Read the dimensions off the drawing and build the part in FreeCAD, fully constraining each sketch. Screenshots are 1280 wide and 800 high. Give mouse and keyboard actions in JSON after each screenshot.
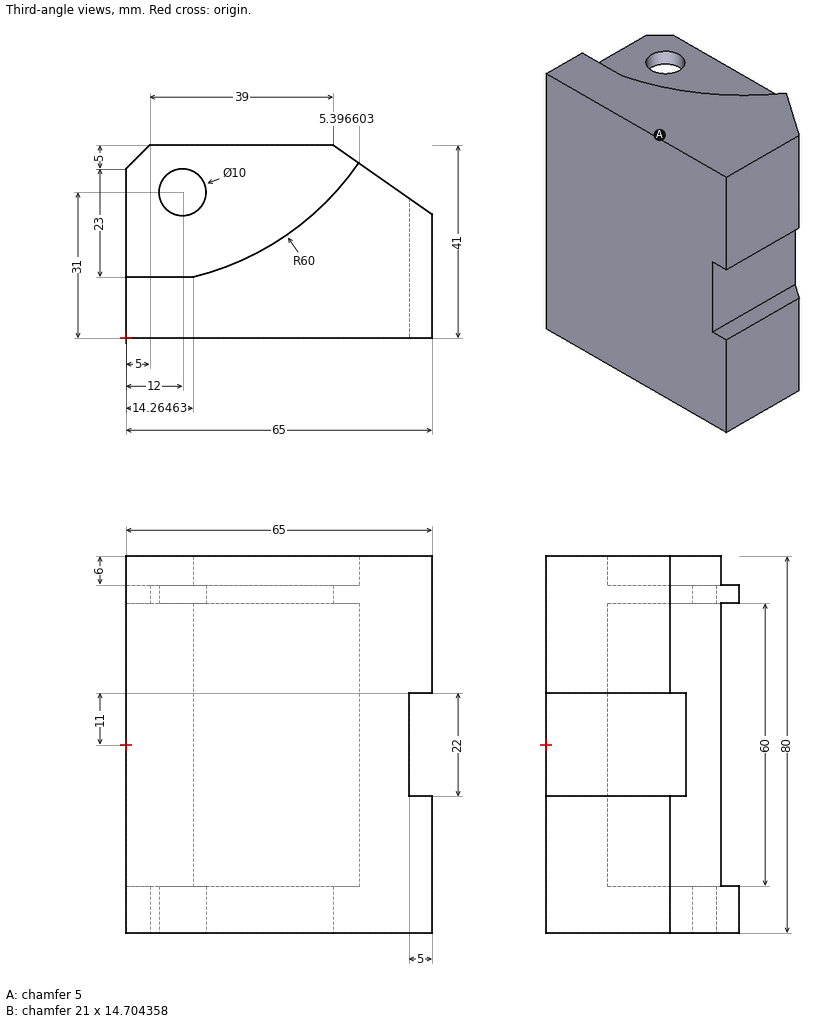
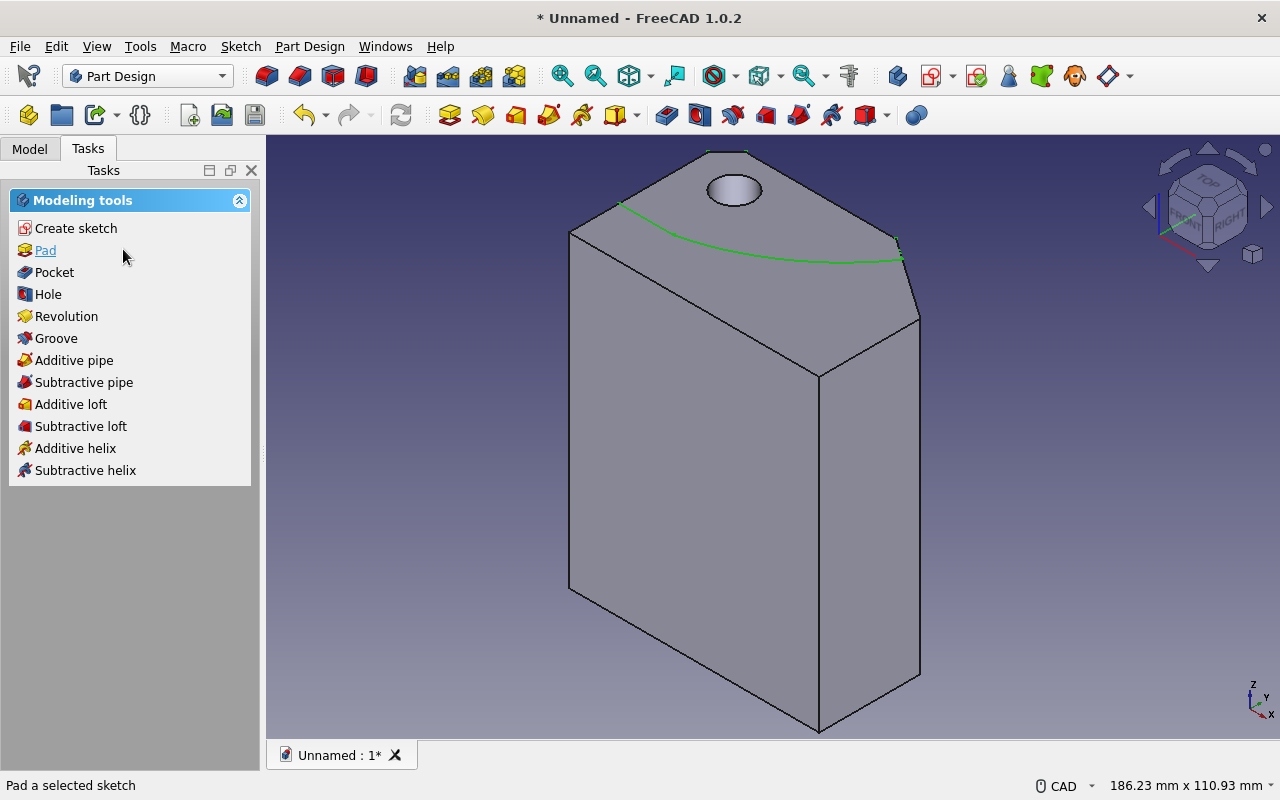
{"action": "left_click", "coordinate": [667, 116]}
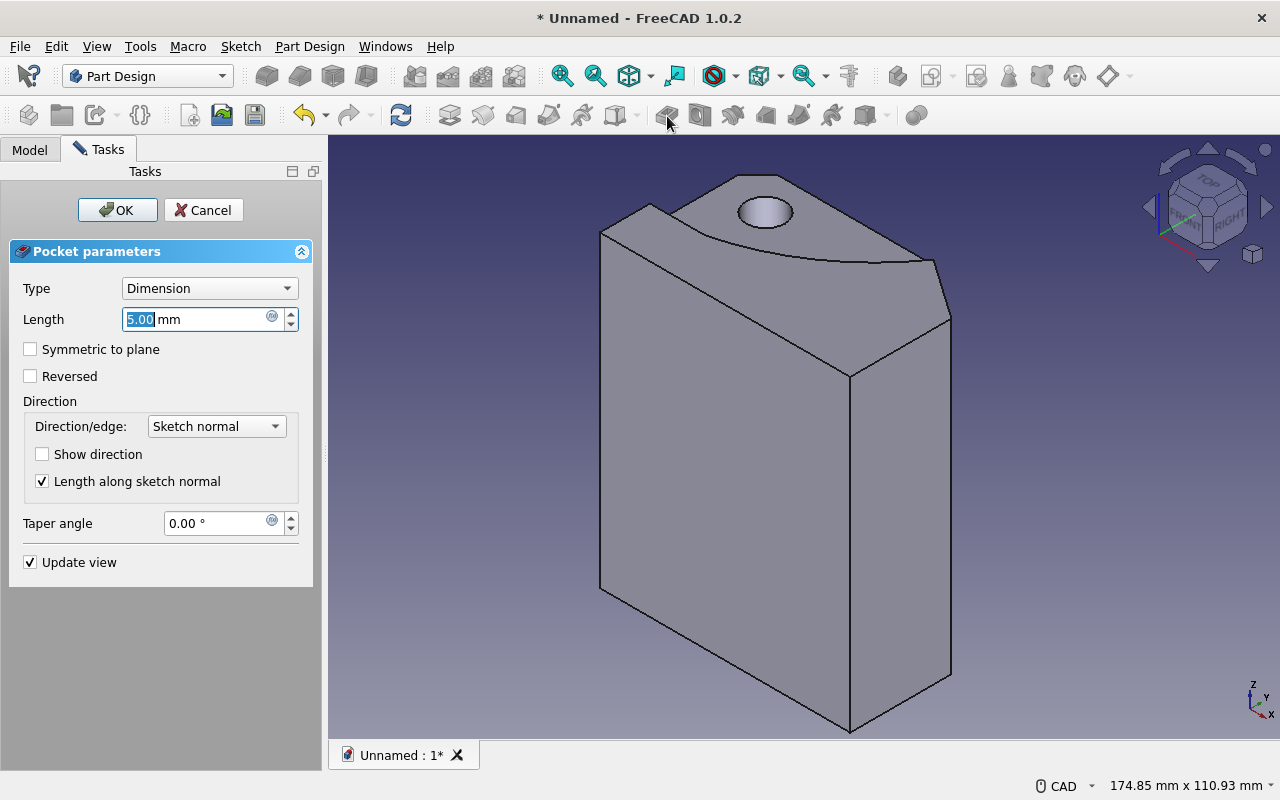
{"action": "type", "text": "6"}
{"action": "key", "text": "Tab"}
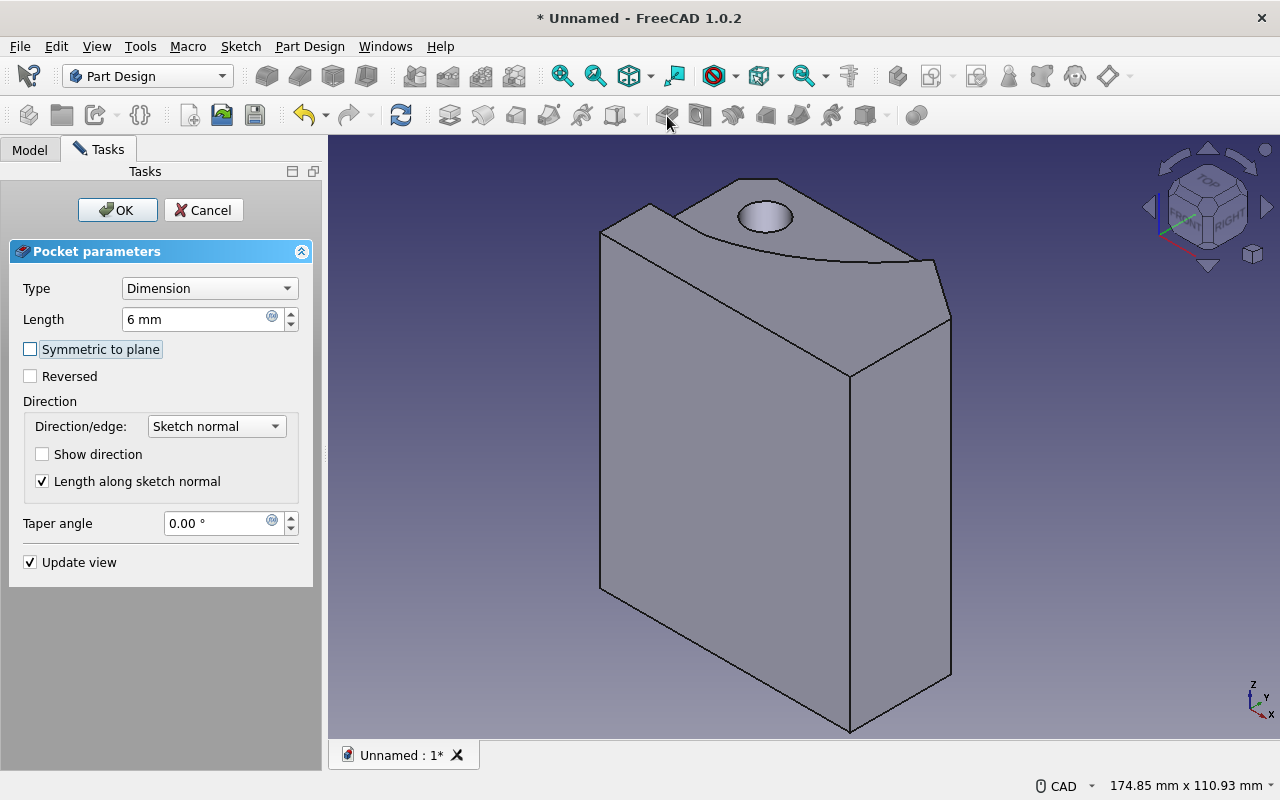
{"action": "left_click", "coordinate": [118, 210]}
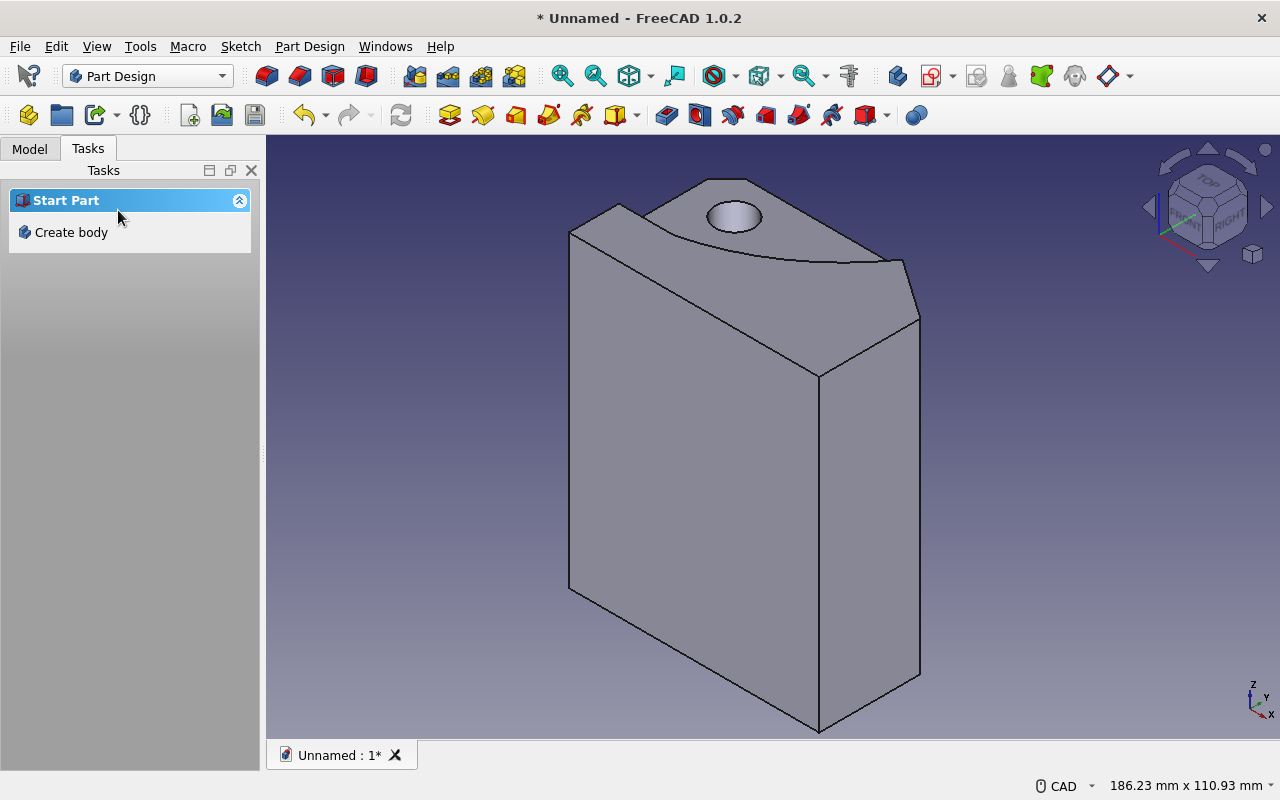
{"action": "left_click", "coordinate": [30, 148]}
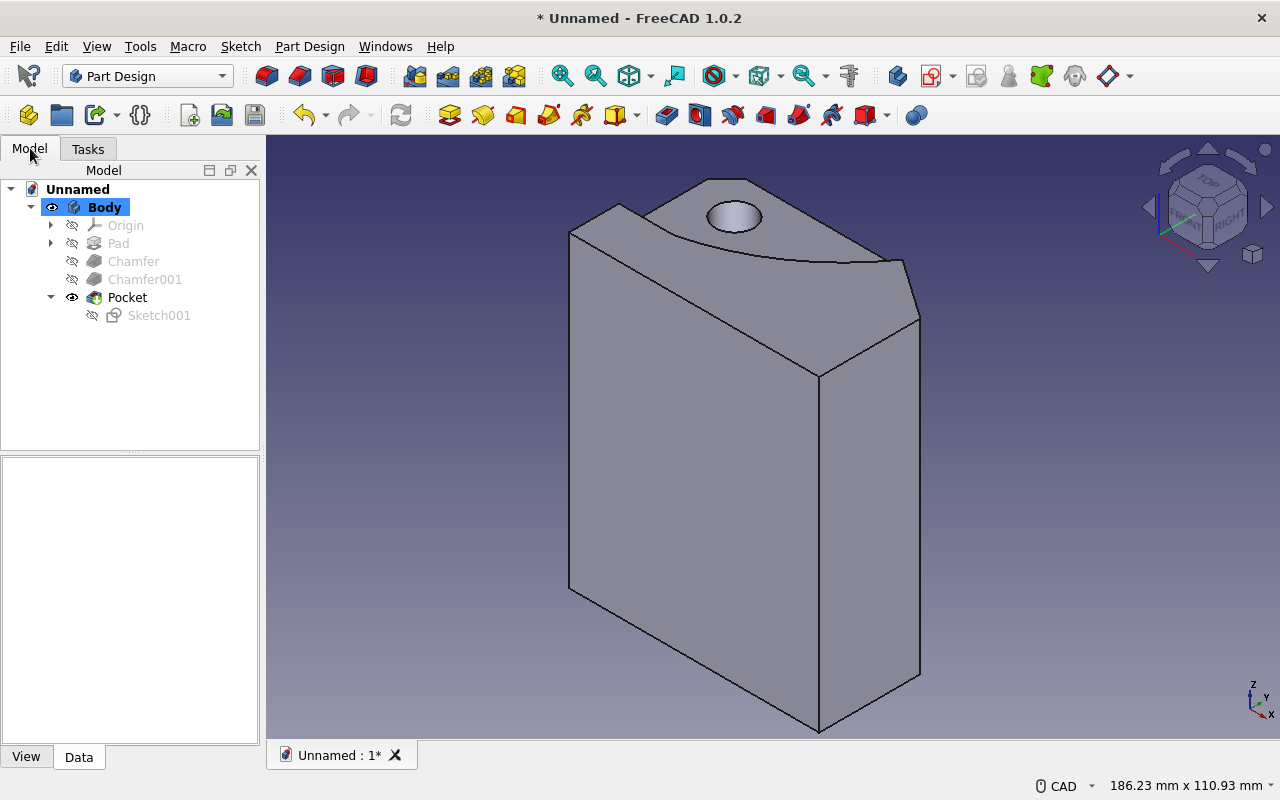
{"action": "left_click", "coordinate": [51, 225]}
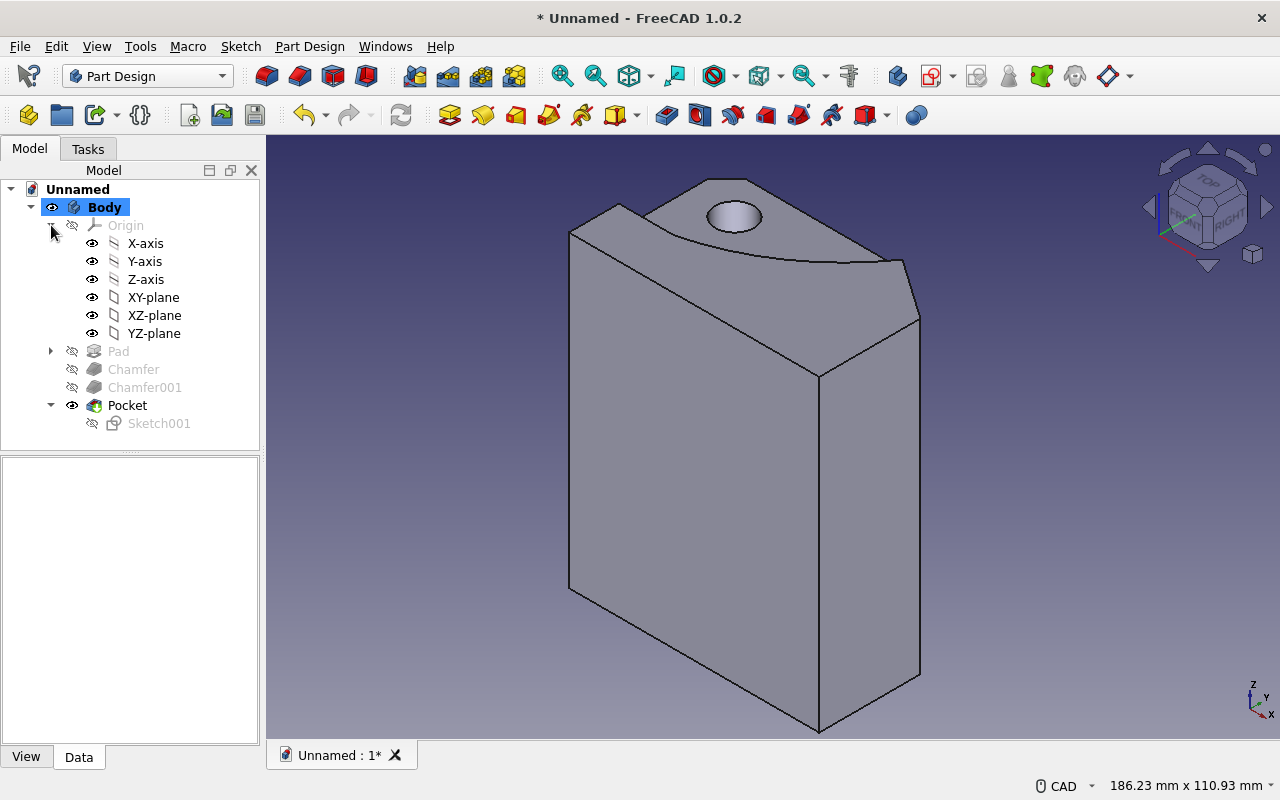
{"action": "left_click", "coordinate": [137, 297]}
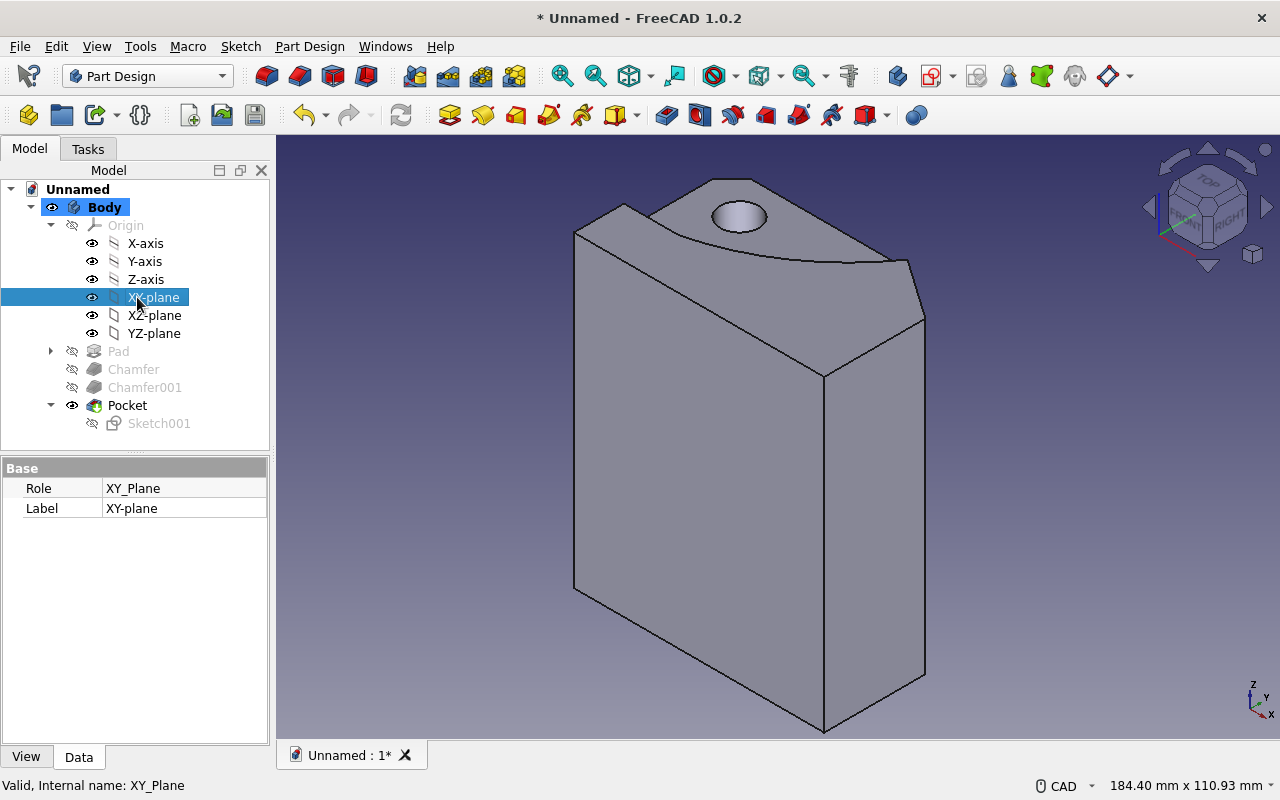
{"action": "left_click", "coordinate": [1108, 76]}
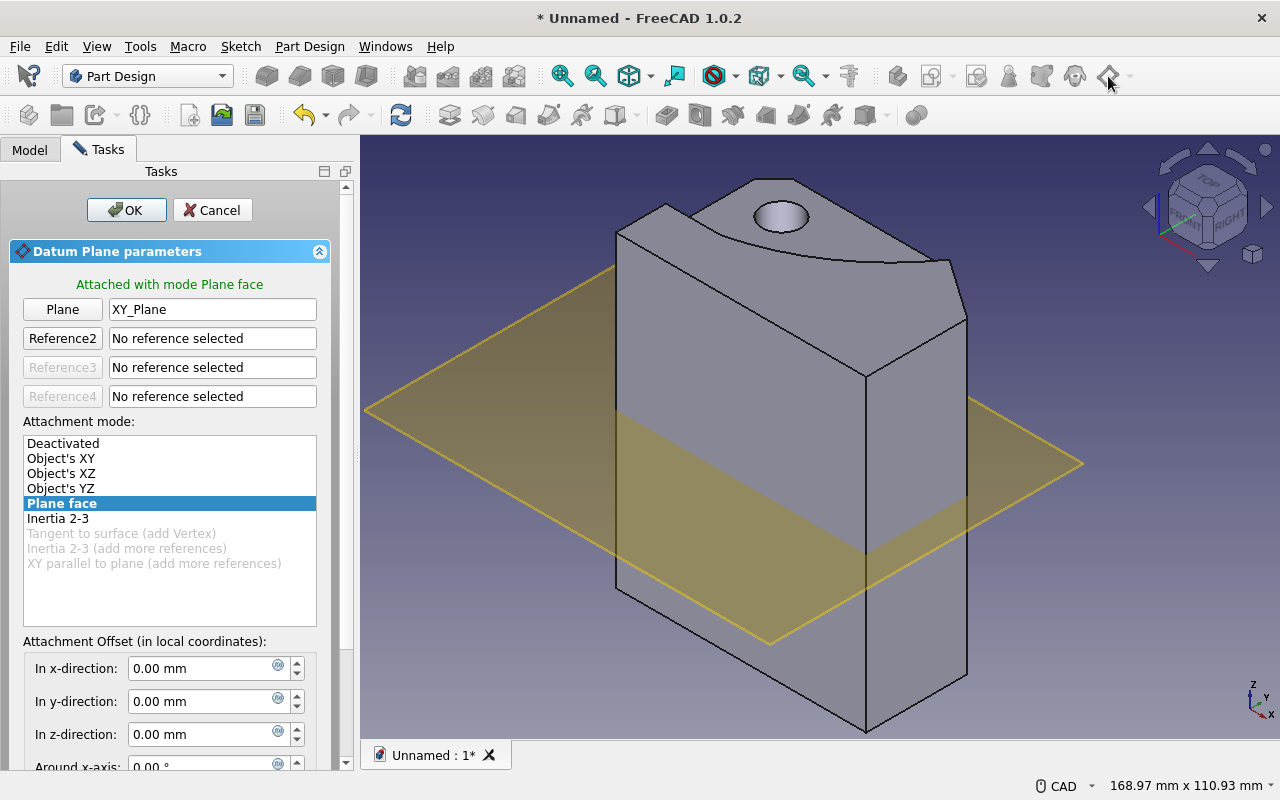
{"action": "triple_click", "coordinate": [210, 734]}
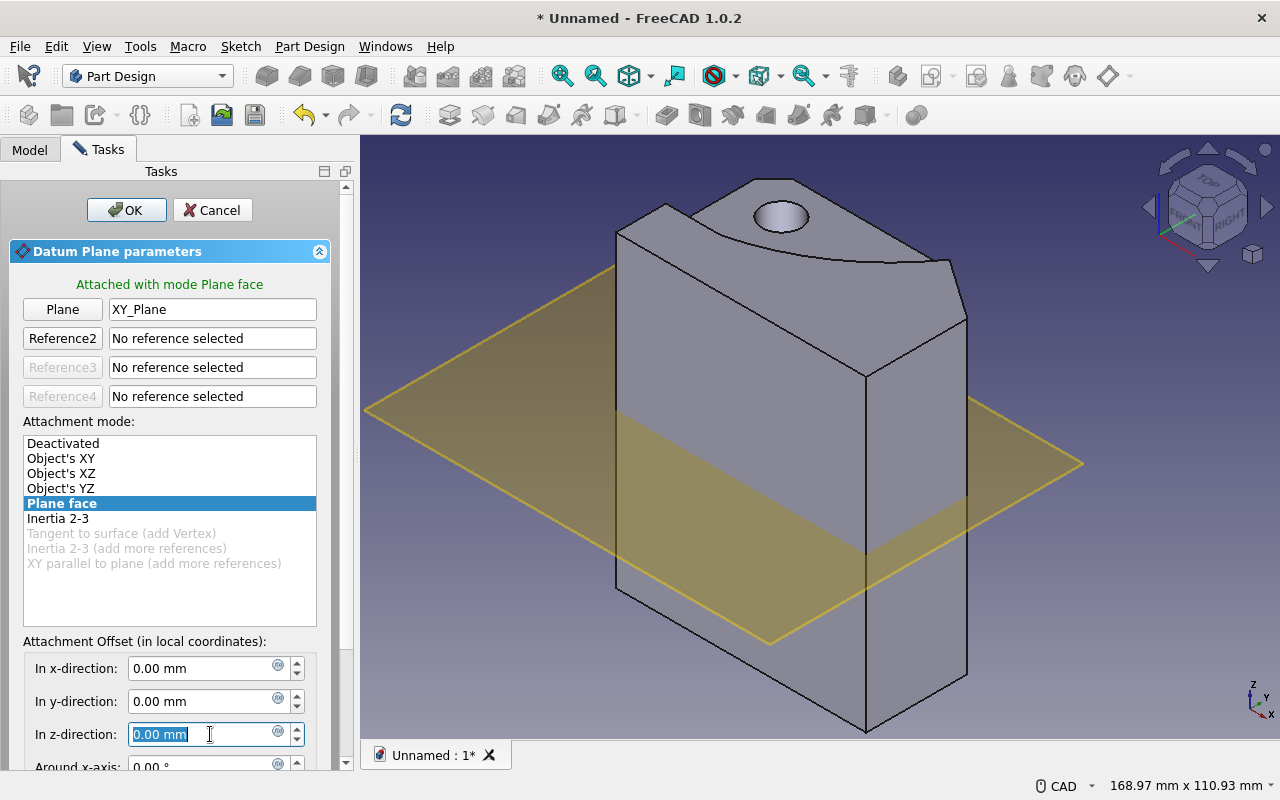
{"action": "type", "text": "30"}
{"action": "key", "text": "Tab"}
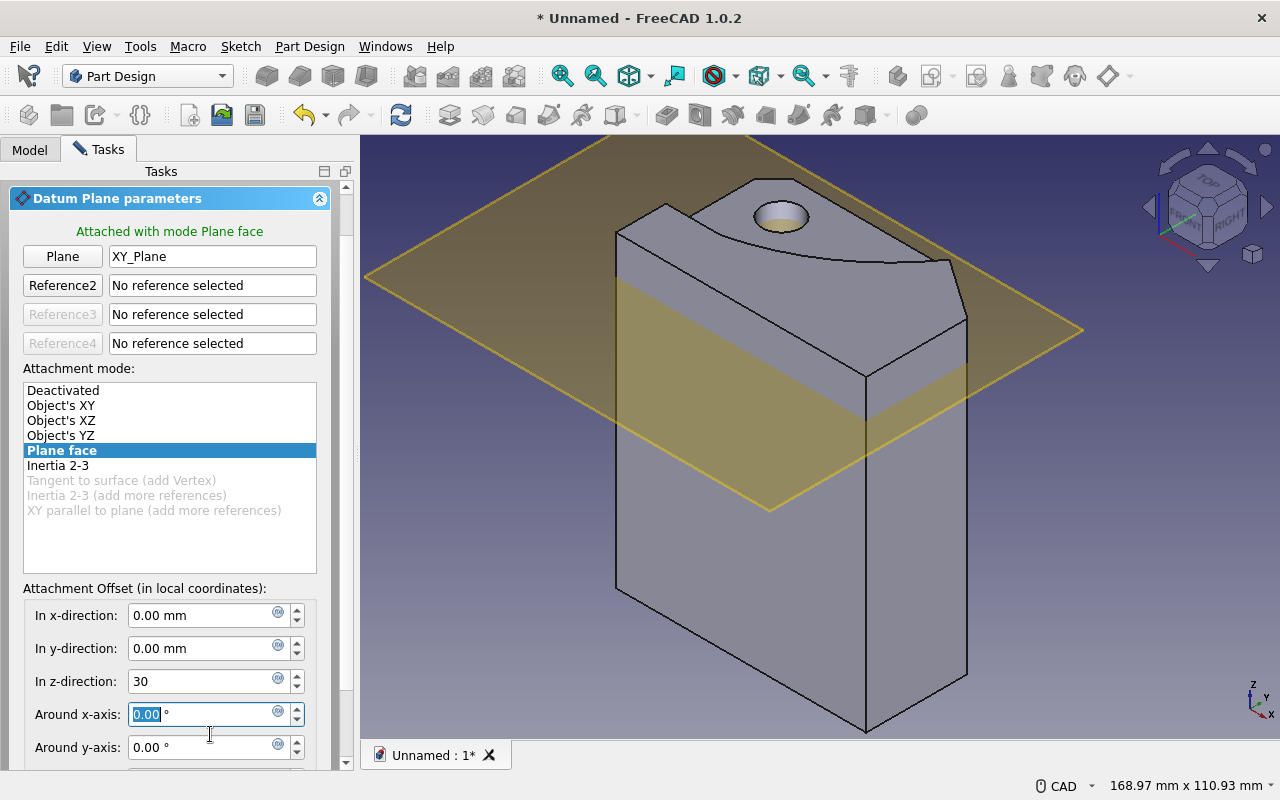
{"action": "scroll", "coordinate": [346, 476], "scroll_direction": "up", "scroll_amount": 2}